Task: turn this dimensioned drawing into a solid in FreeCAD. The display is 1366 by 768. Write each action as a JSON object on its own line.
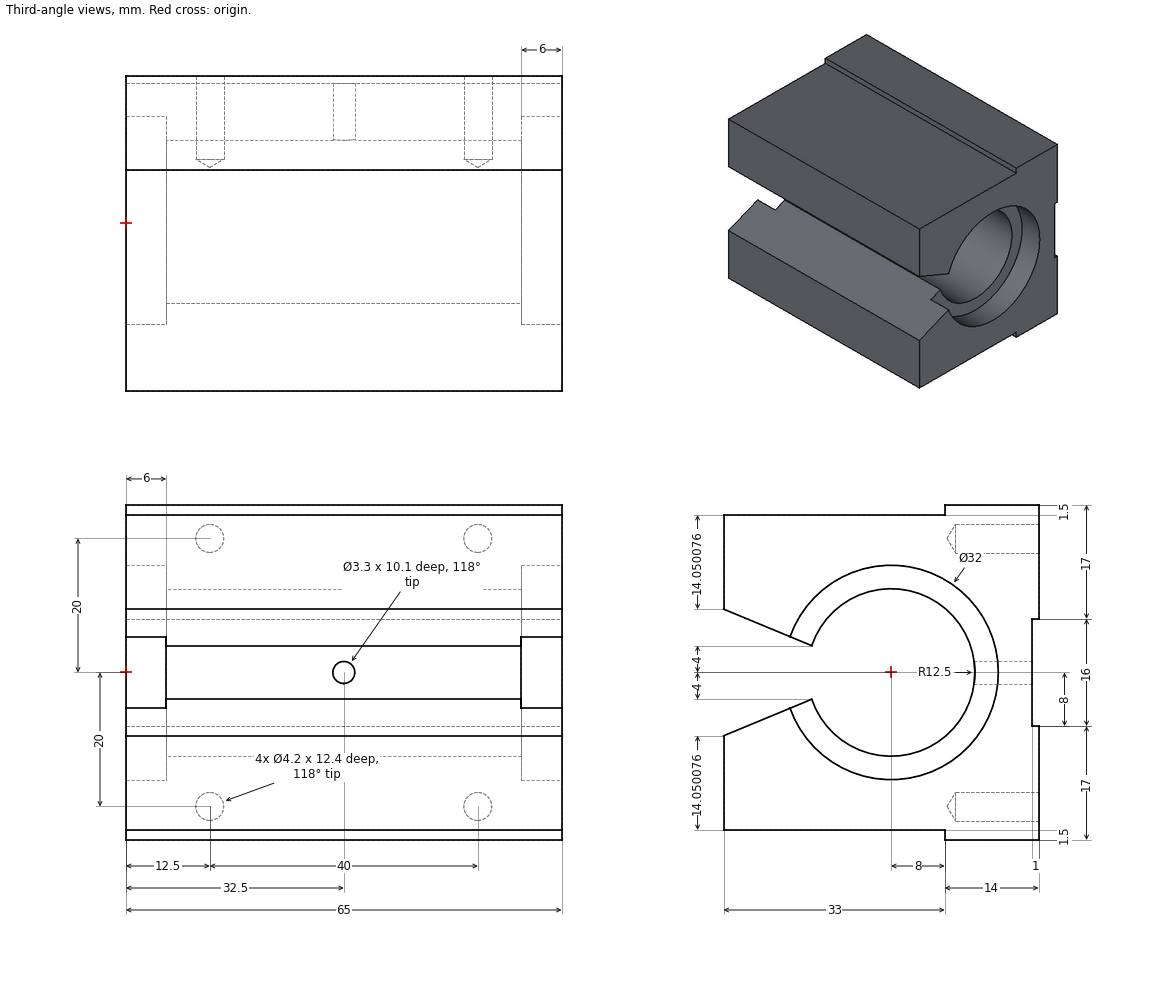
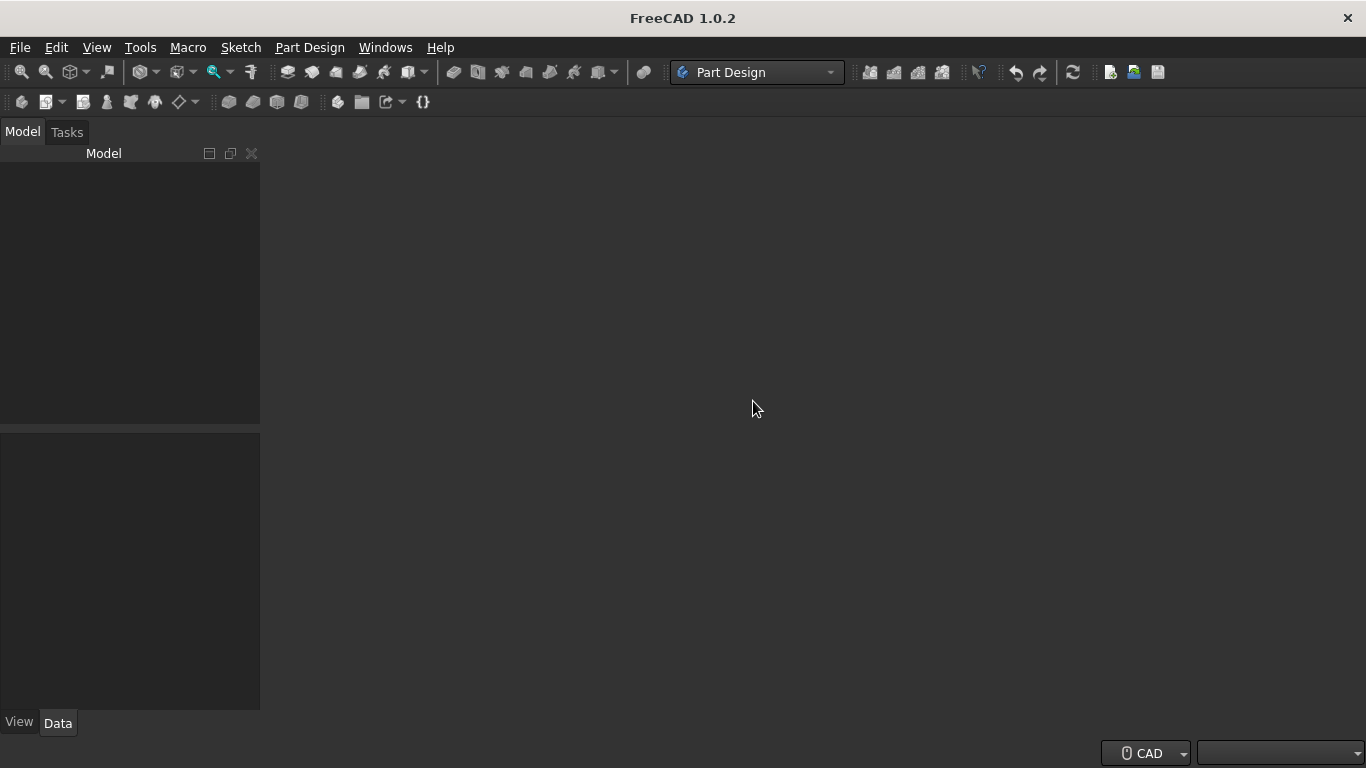
{"action": "key", "text": "ctrl+n"}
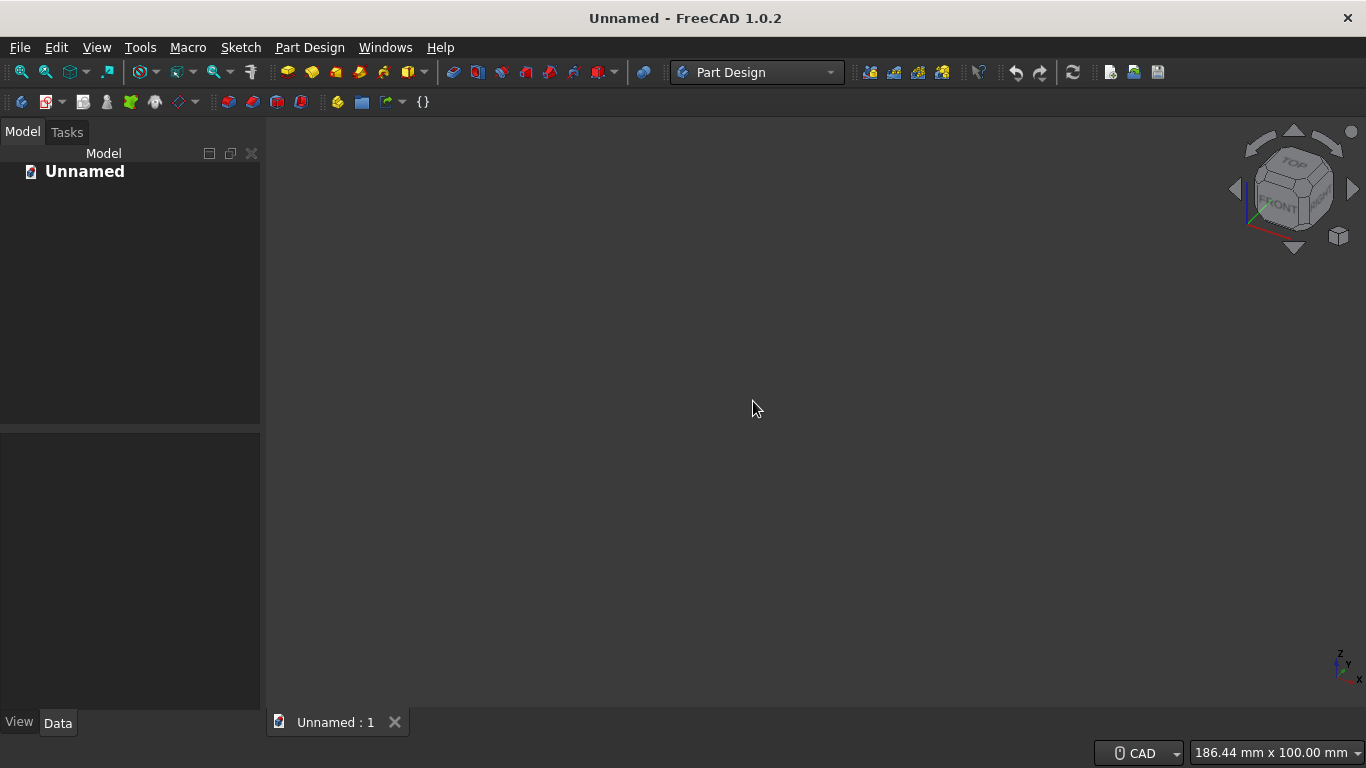
{"action": "left_click", "coordinate": [46, 102]}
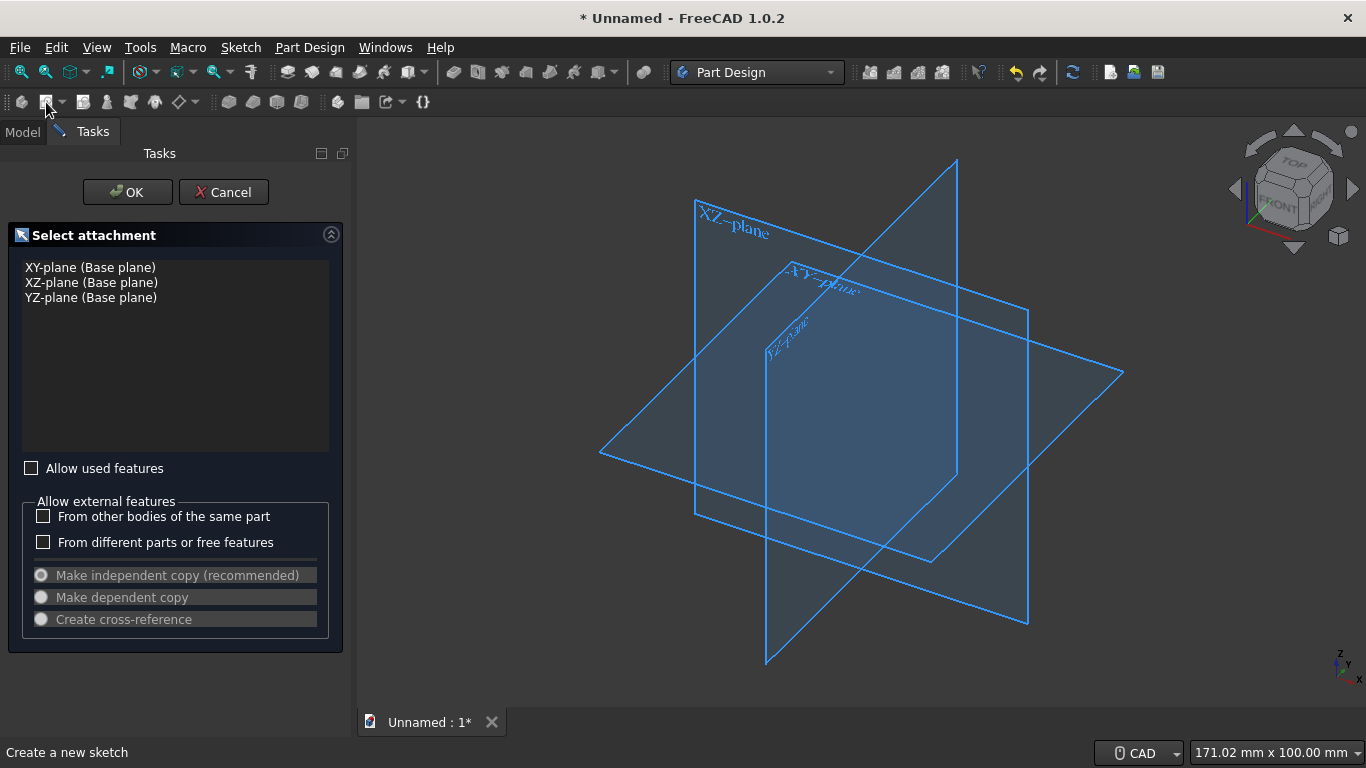
{"action": "left_click", "coordinate": [82, 298]}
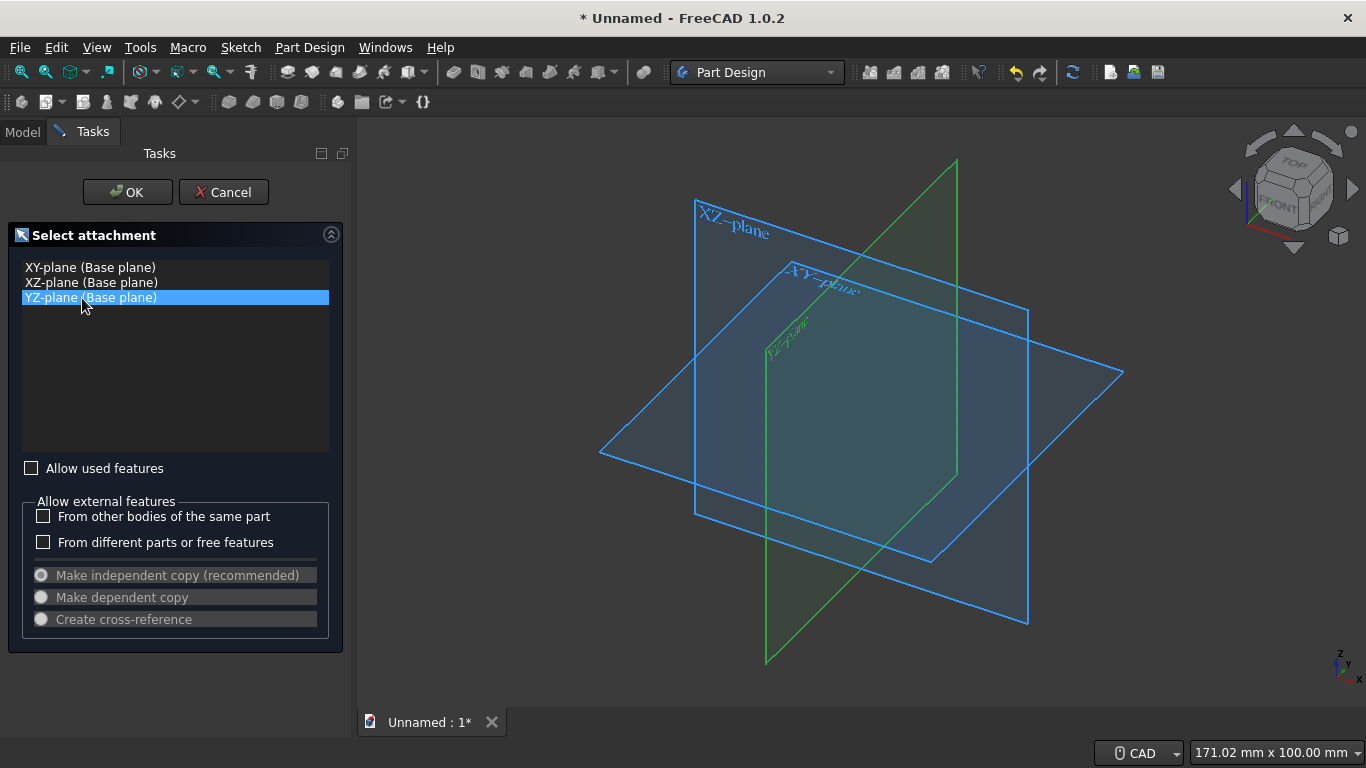
{"action": "left_click", "coordinate": [128, 192]}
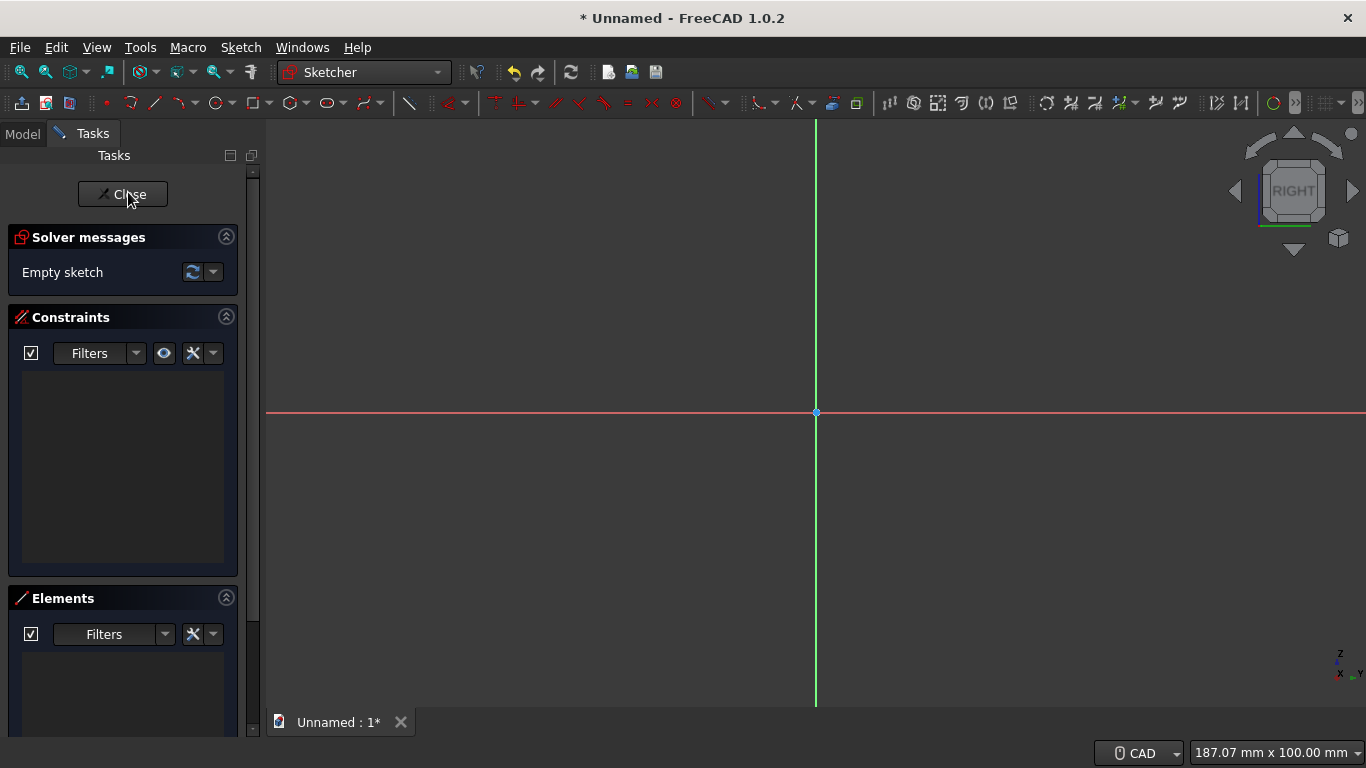
{"action": "left_click", "coordinate": [132, 104]}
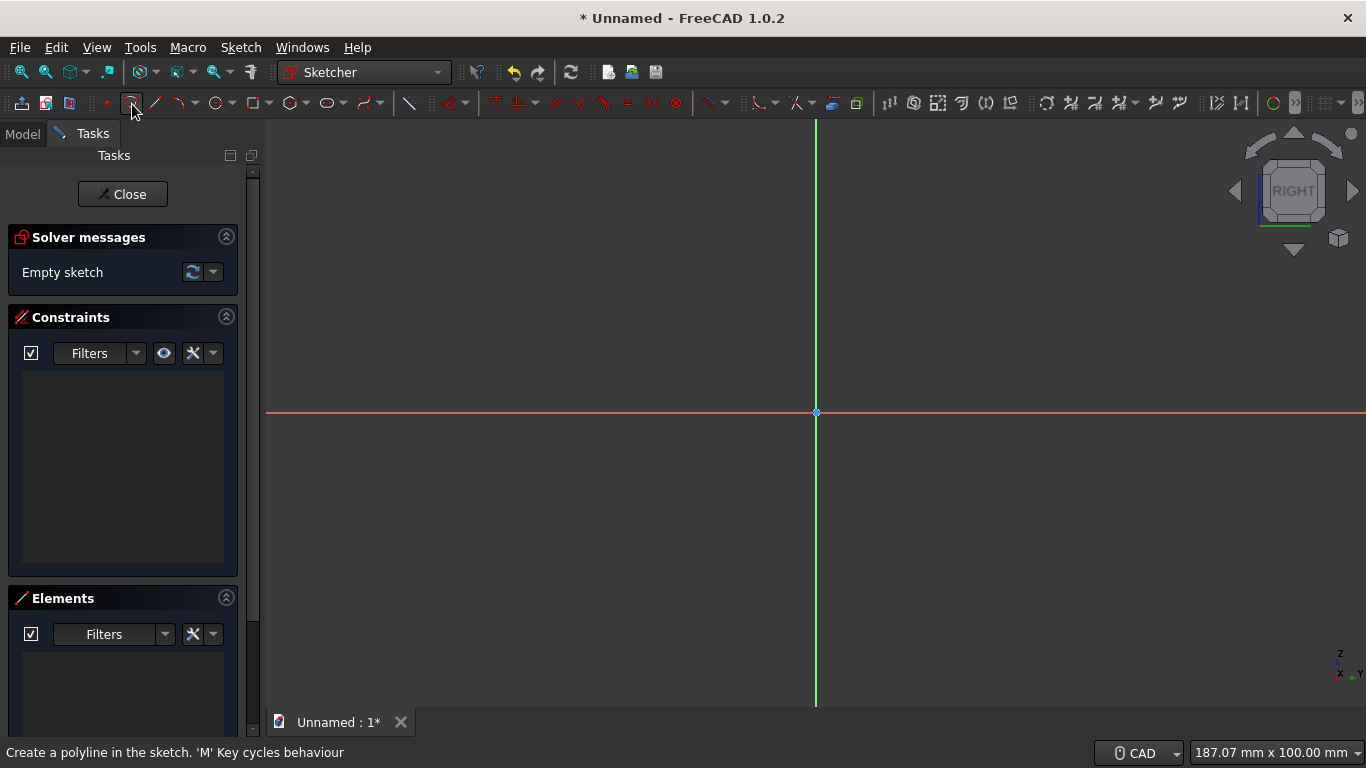
{"action": "left_click", "coordinate": [746, 437]}
{"action": "left_click", "coordinate": [669, 469]}
{"action": "left_click", "coordinate": [669, 551]}
{"action": "left_click", "coordinate": [863, 551]}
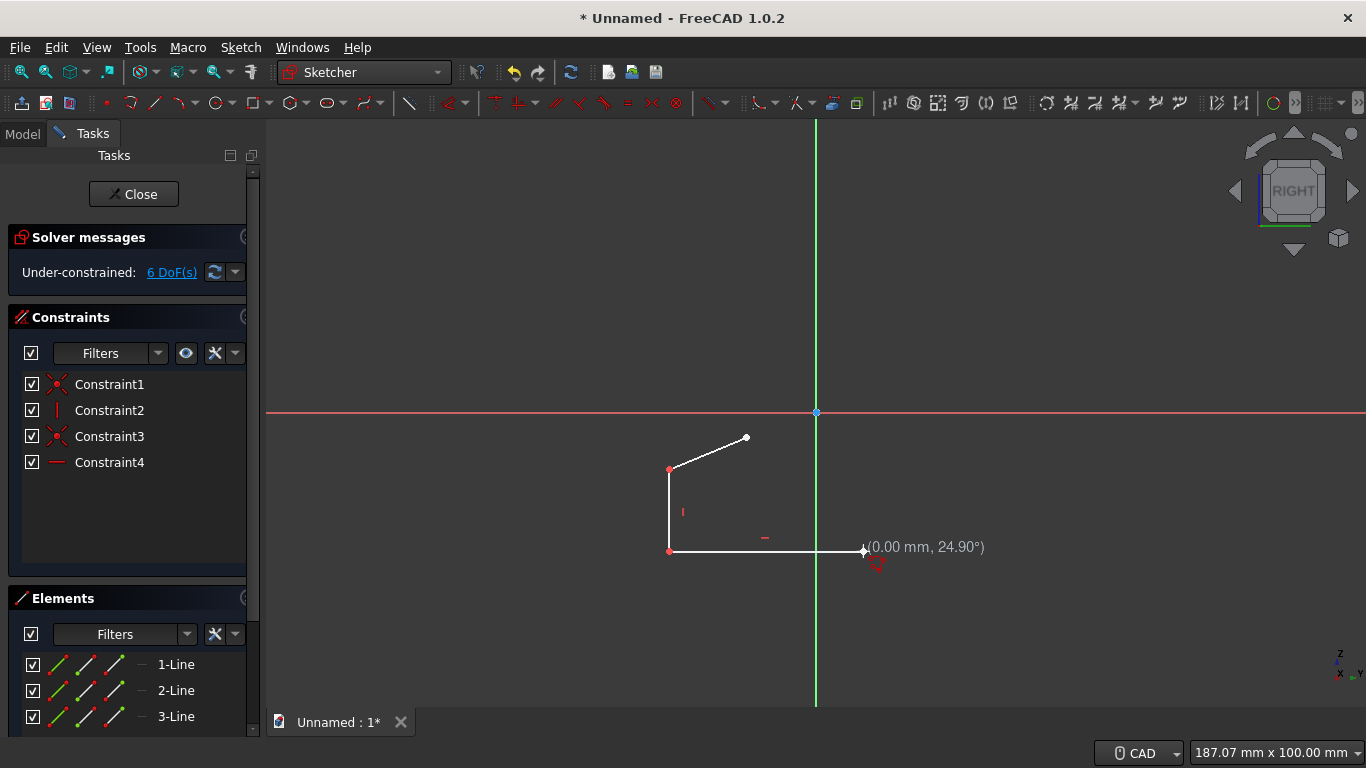
{"action": "scroll", "coordinate": [863, 560], "scroll_direction": "up", "scroll_amount": 3}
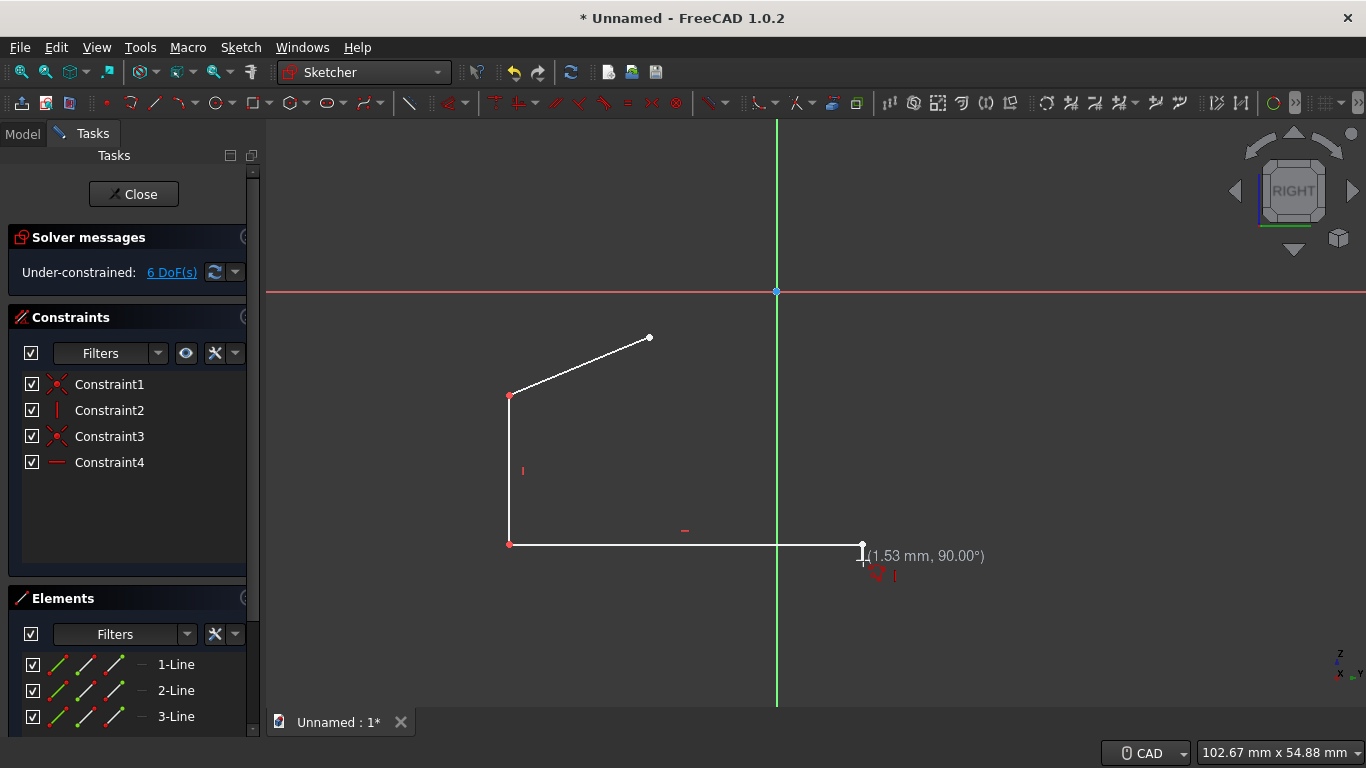
{"action": "left_click", "coordinate": [863, 559]}
{"action": "left_click", "coordinate": [1013, 559]}
{"action": "left_click", "coordinate": [1013, 377]}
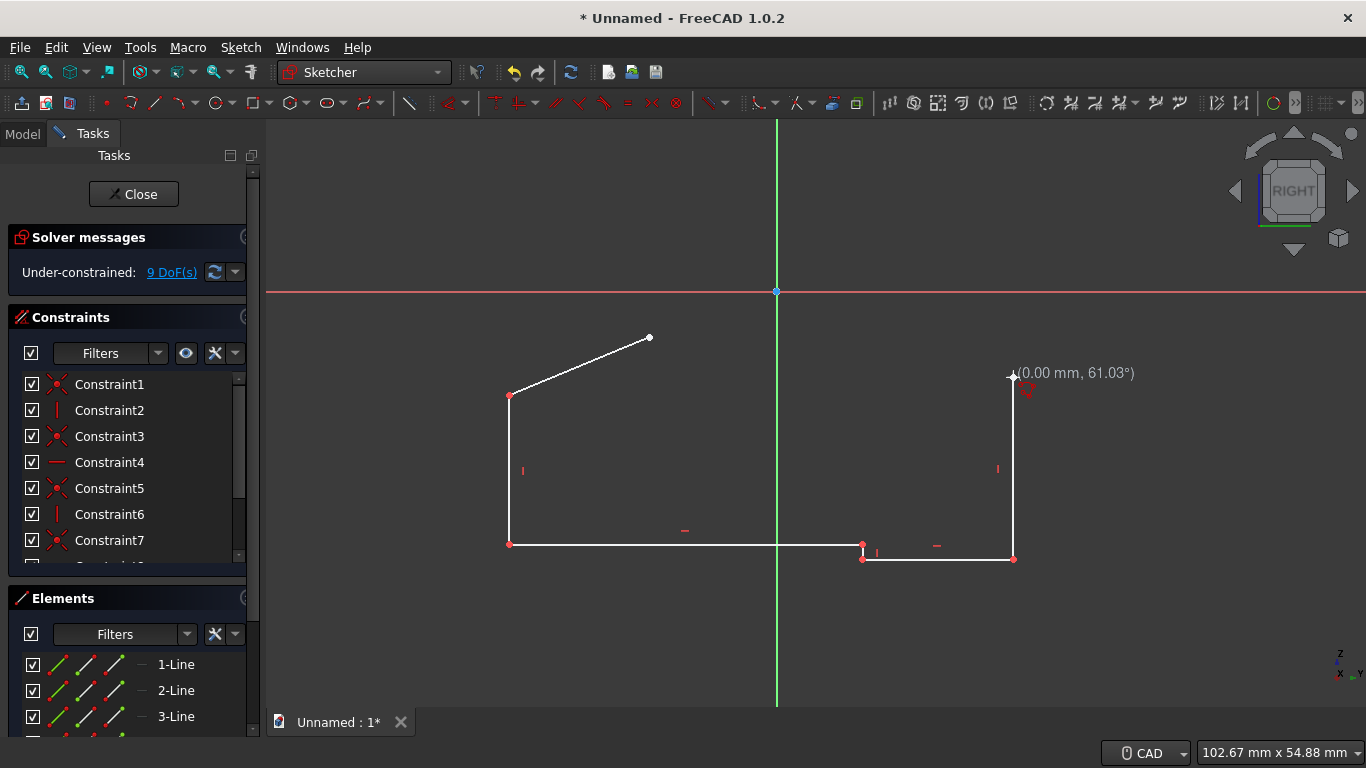
{"action": "scroll", "coordinate": [1002, 377], "scroll_direction": "up", "scroll_amount": 2}